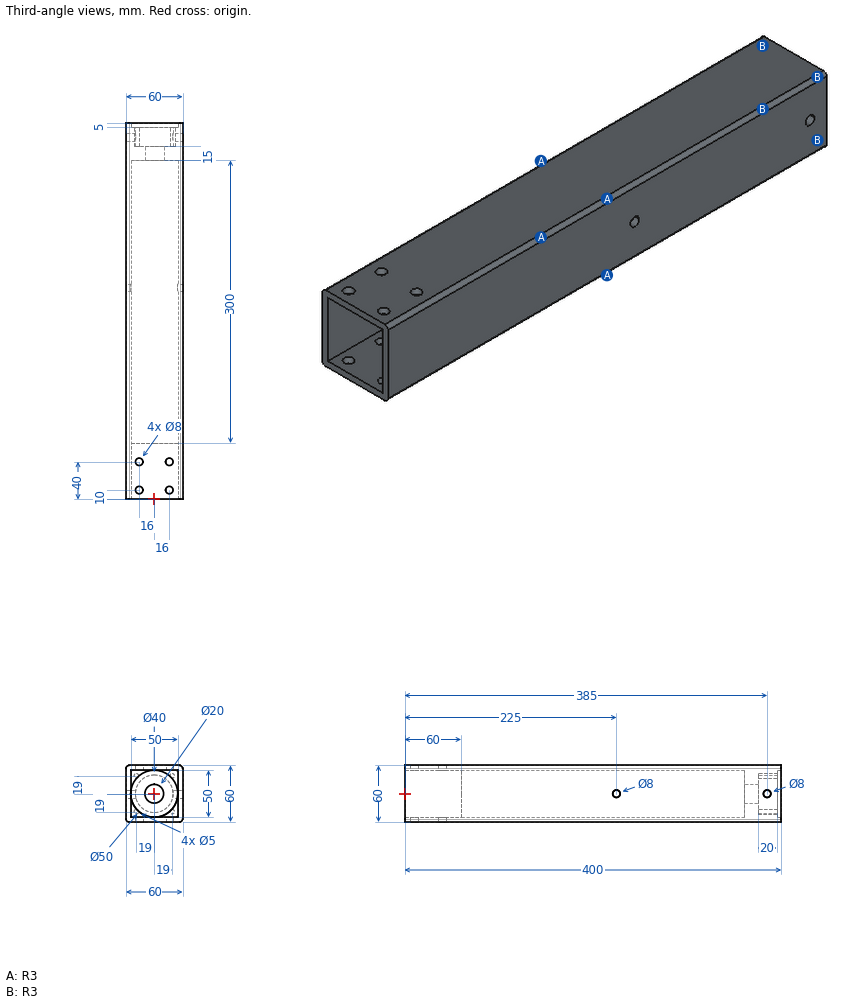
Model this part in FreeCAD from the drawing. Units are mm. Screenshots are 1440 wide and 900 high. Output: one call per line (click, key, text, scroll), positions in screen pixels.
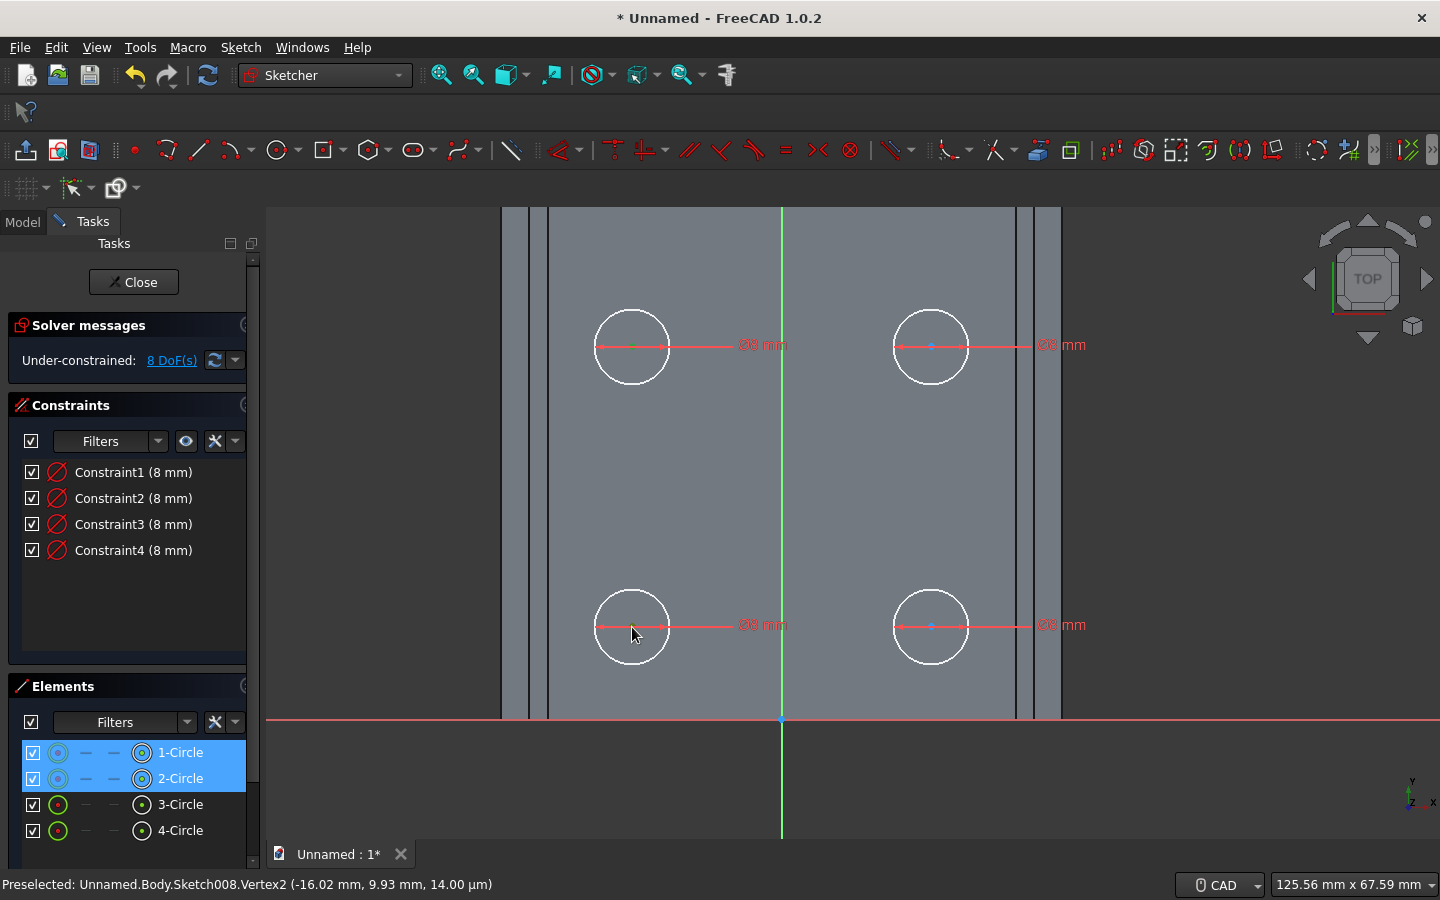
click(668, 150)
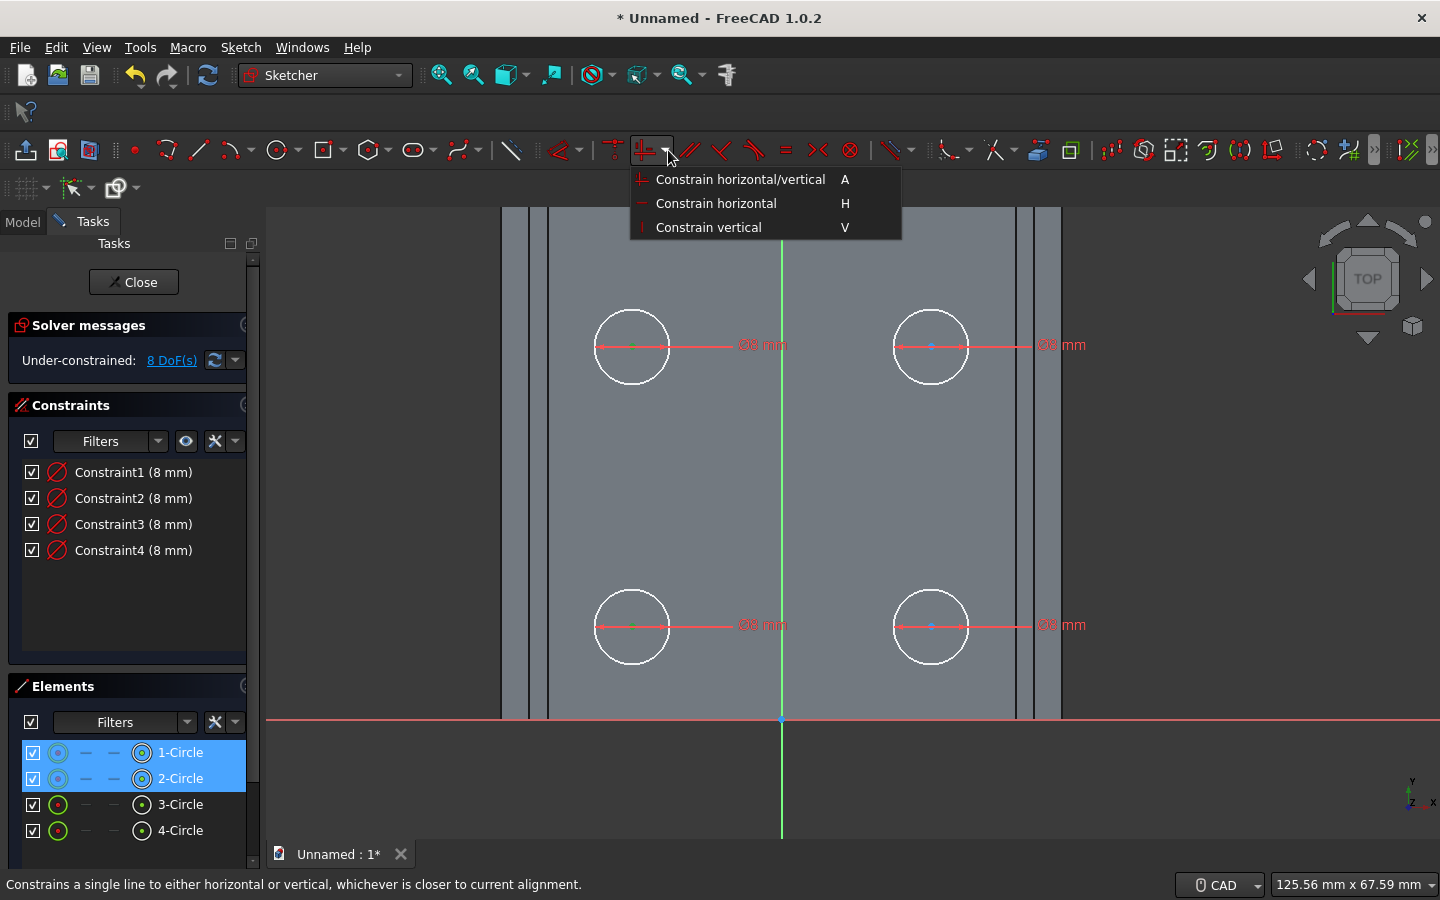
click(766, 227)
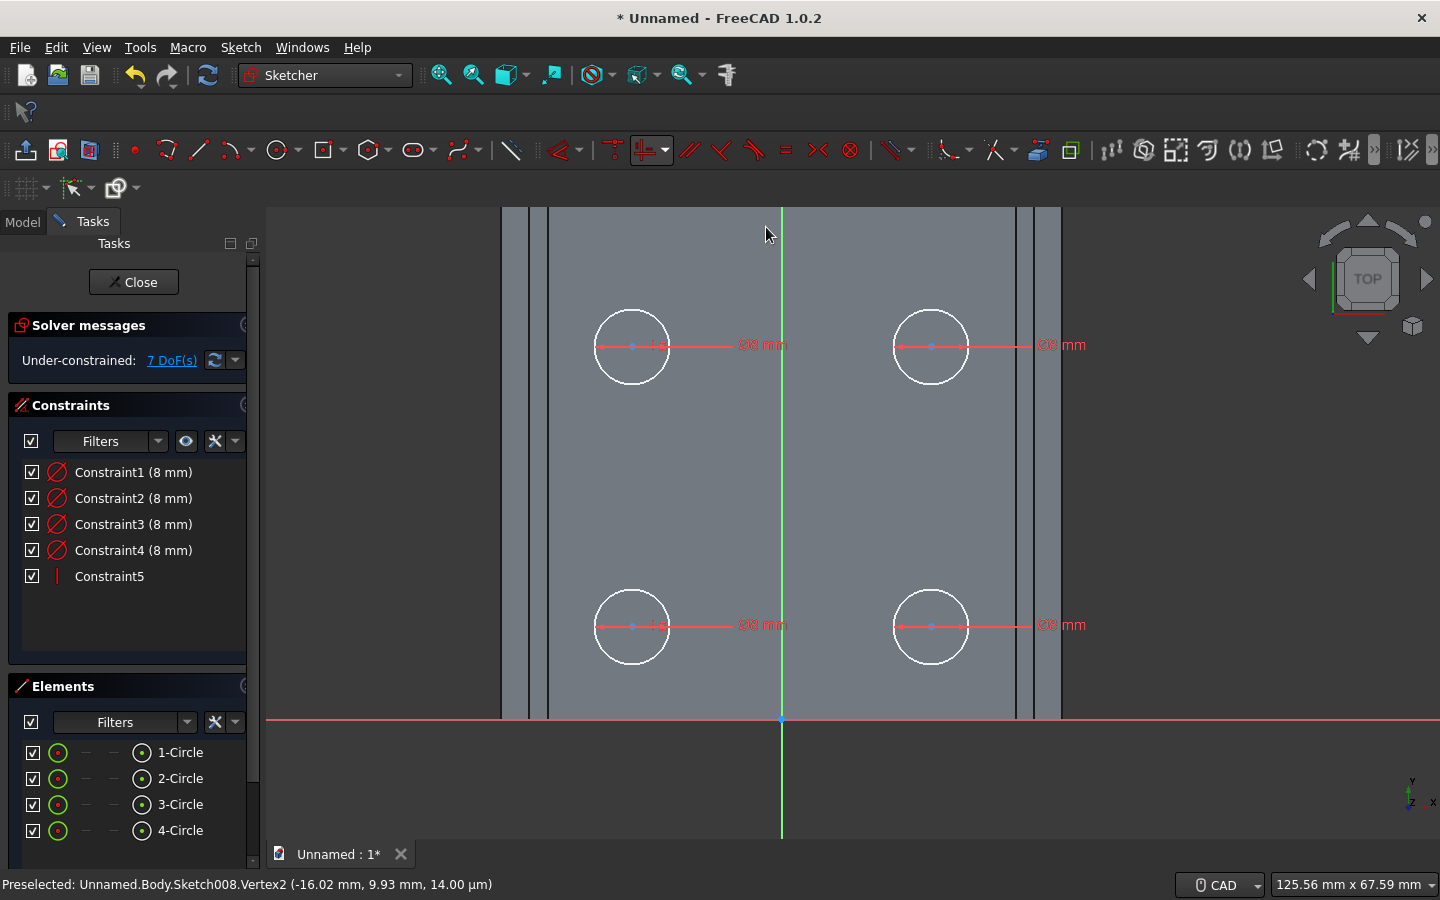
click(632, 627)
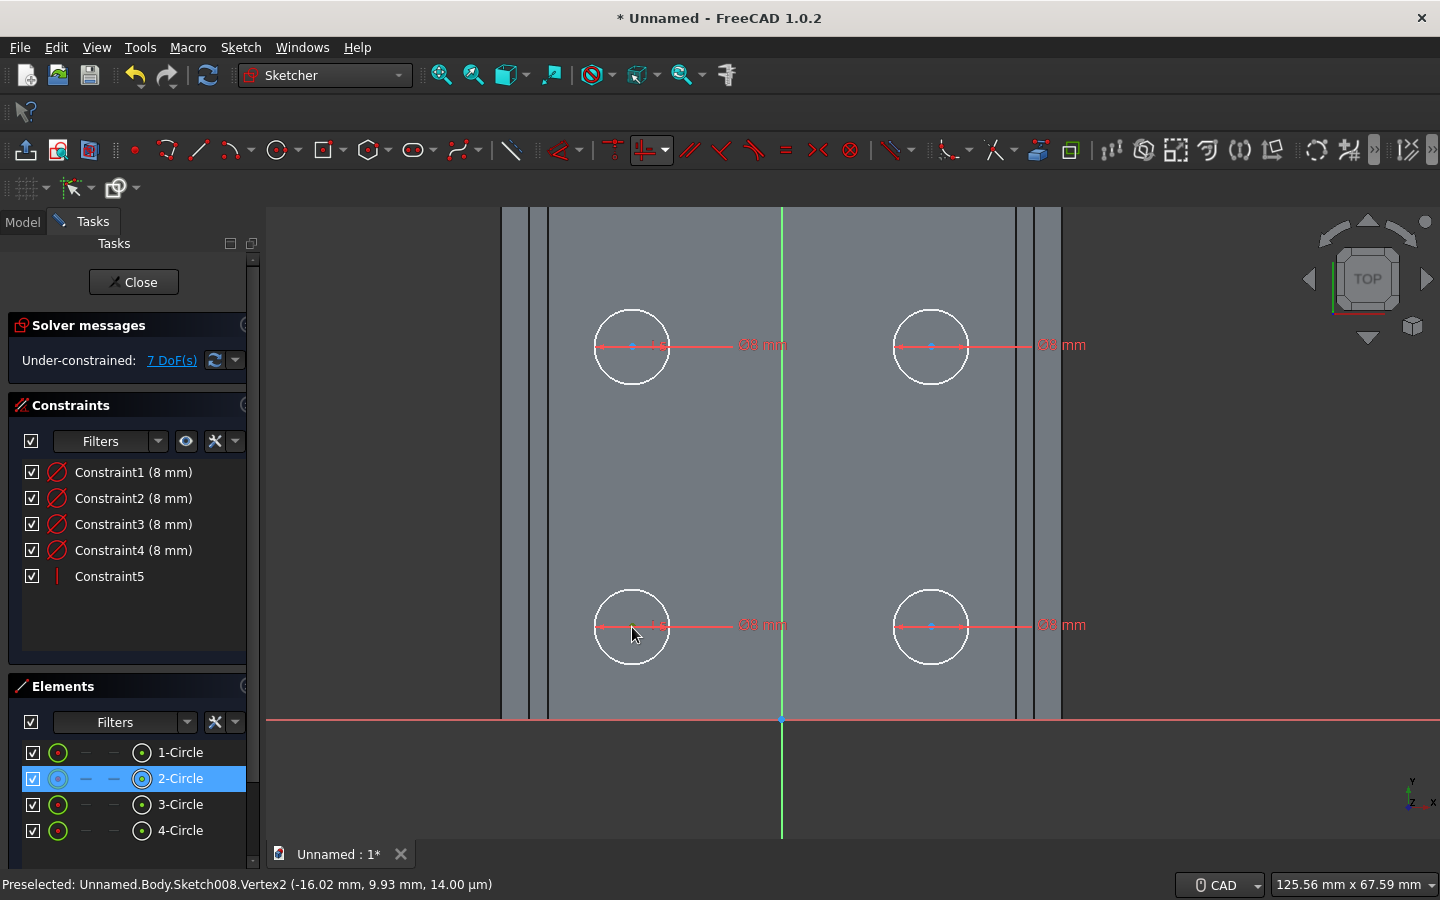
click(931, 627)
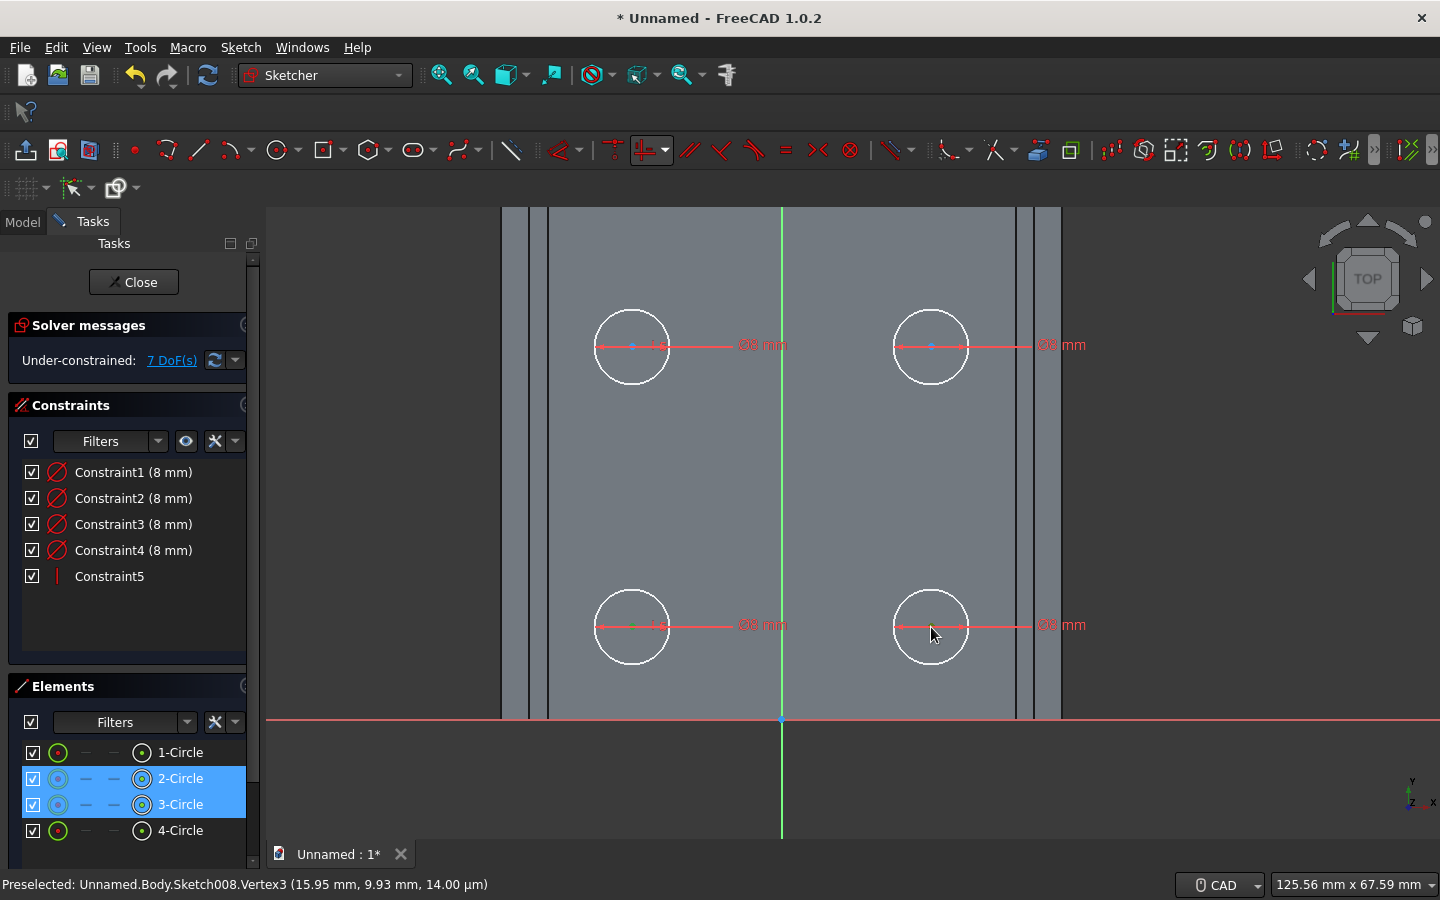
key(h)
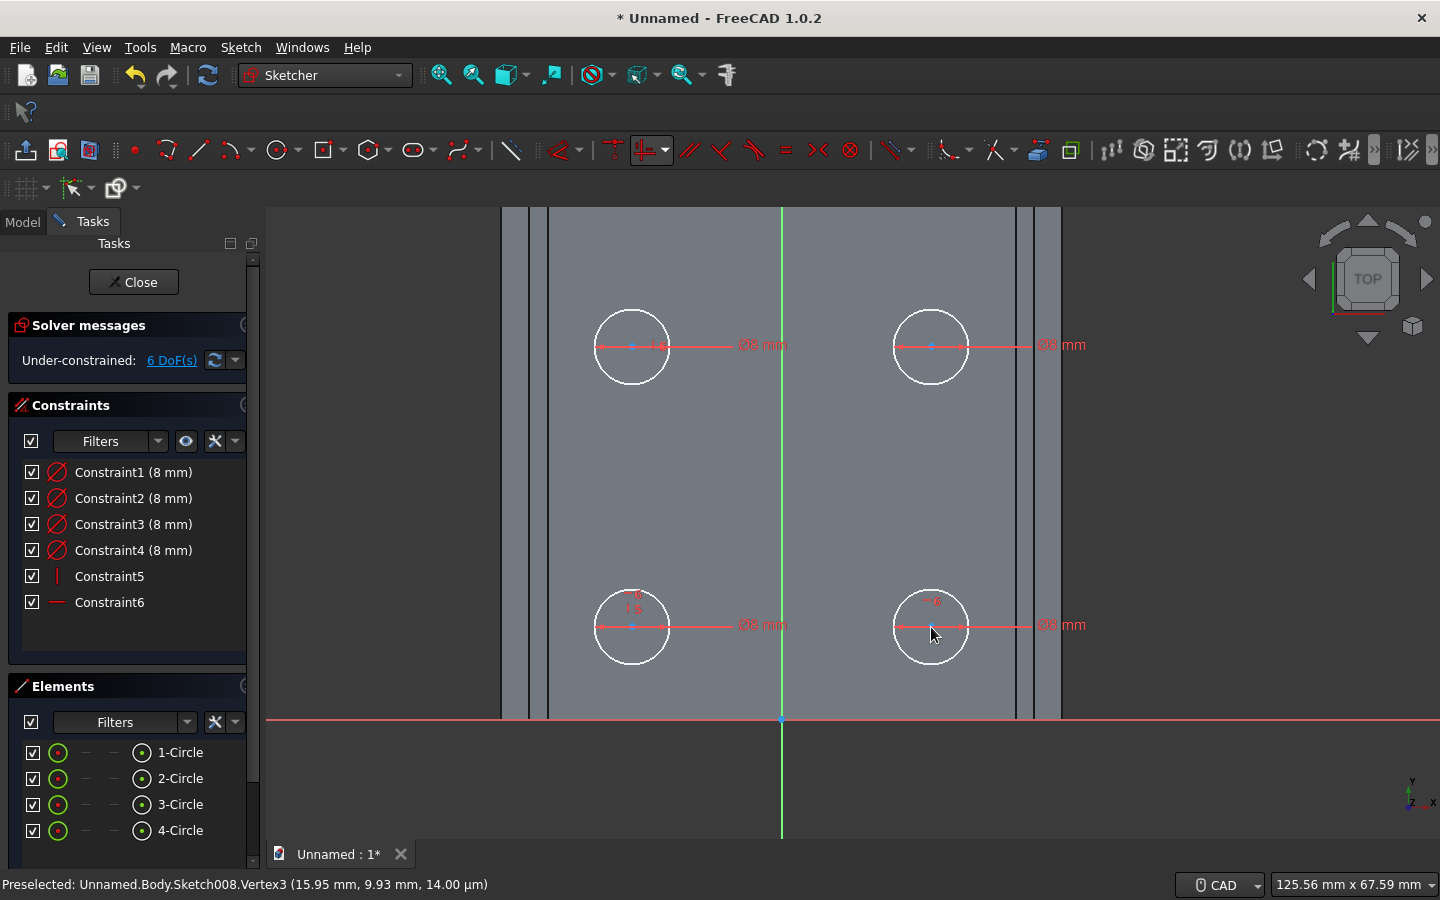
click(931, 627)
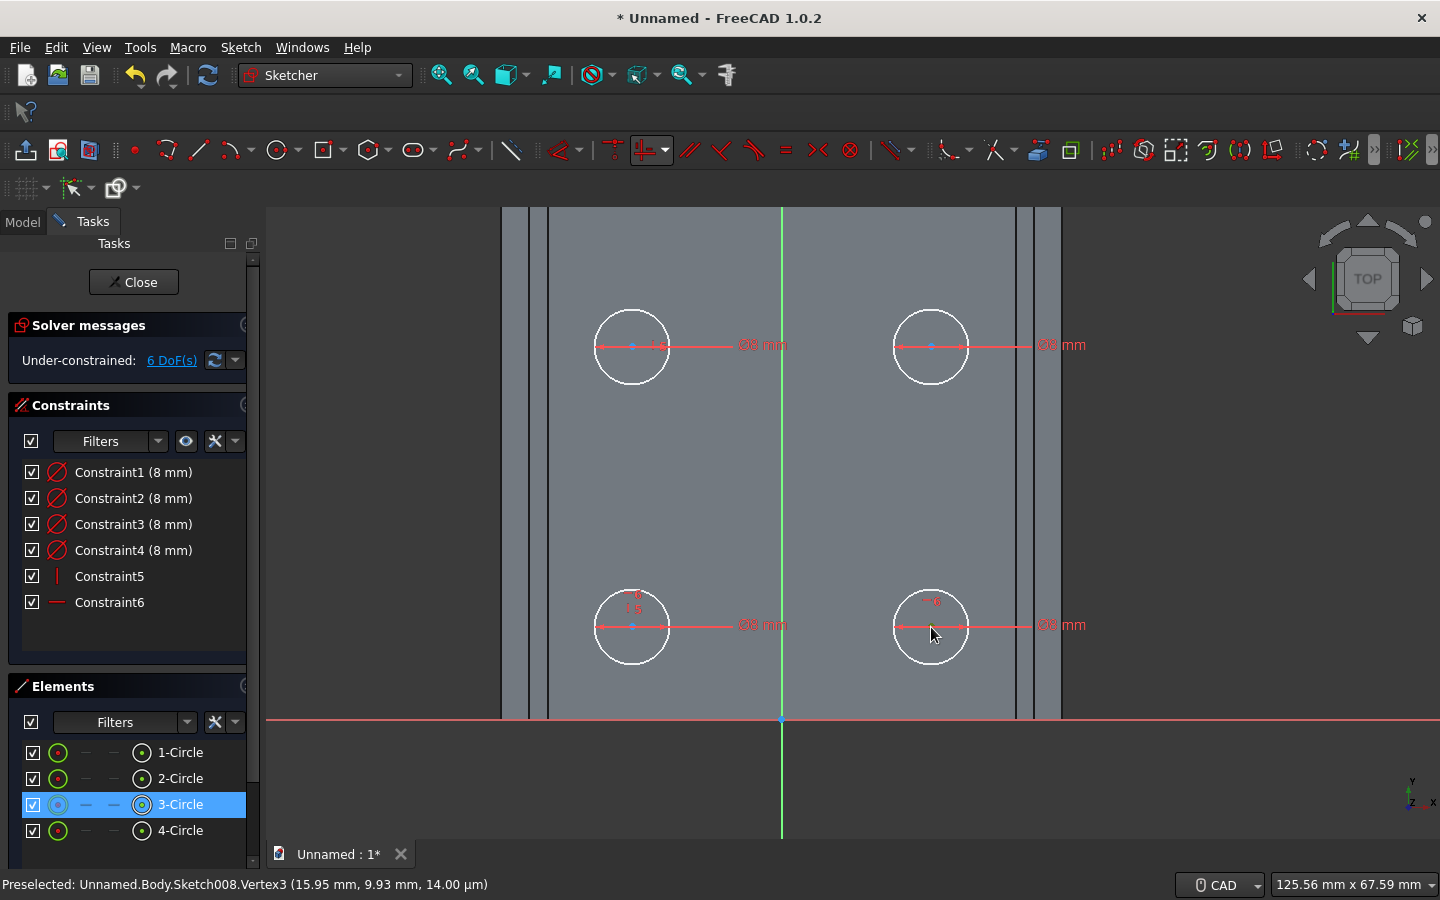
click(931, 347)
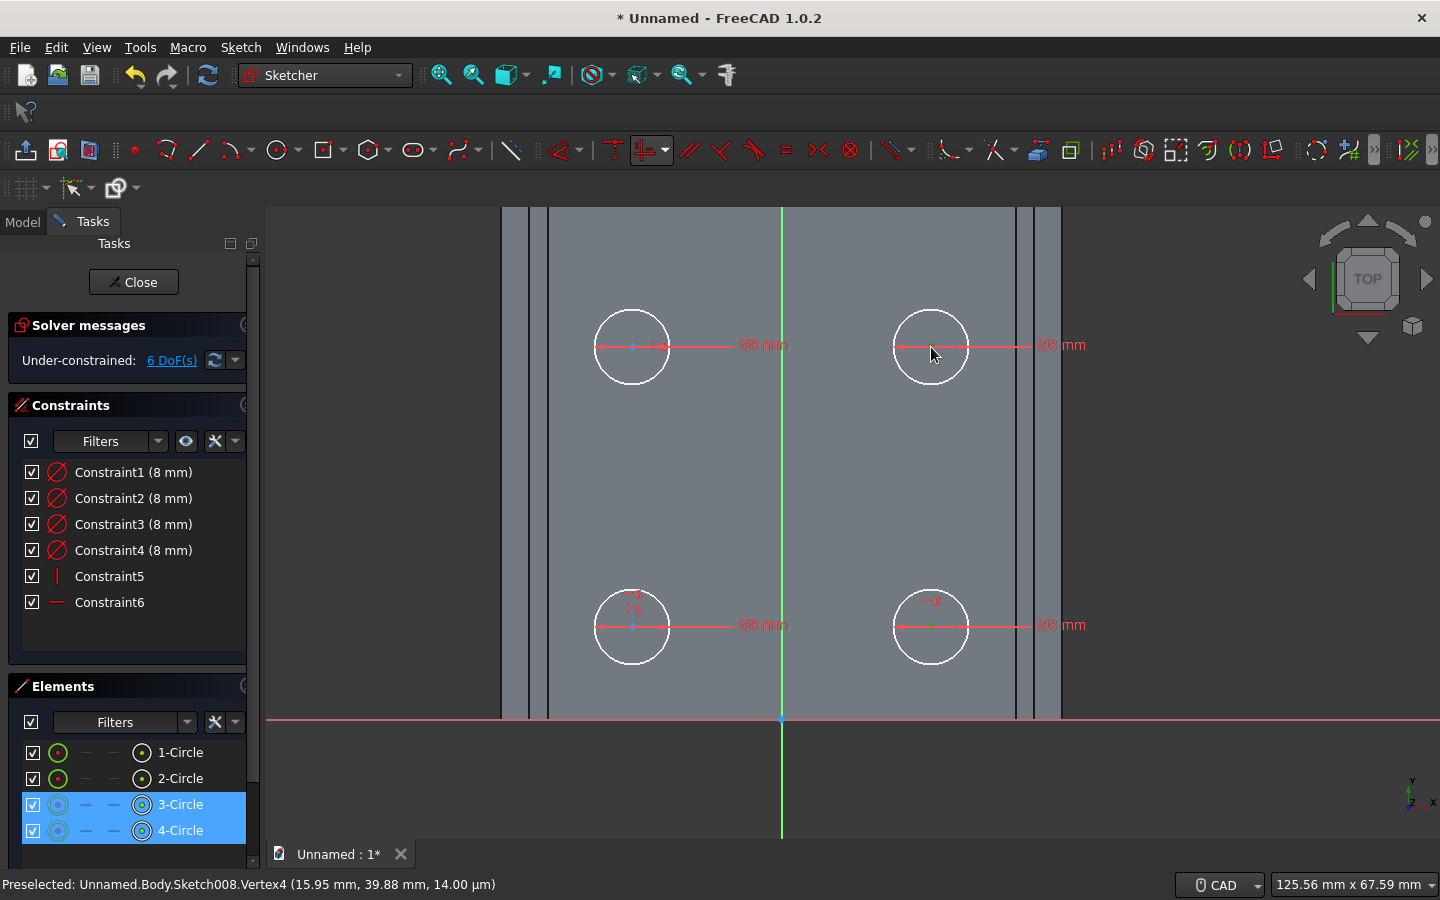
key(v)